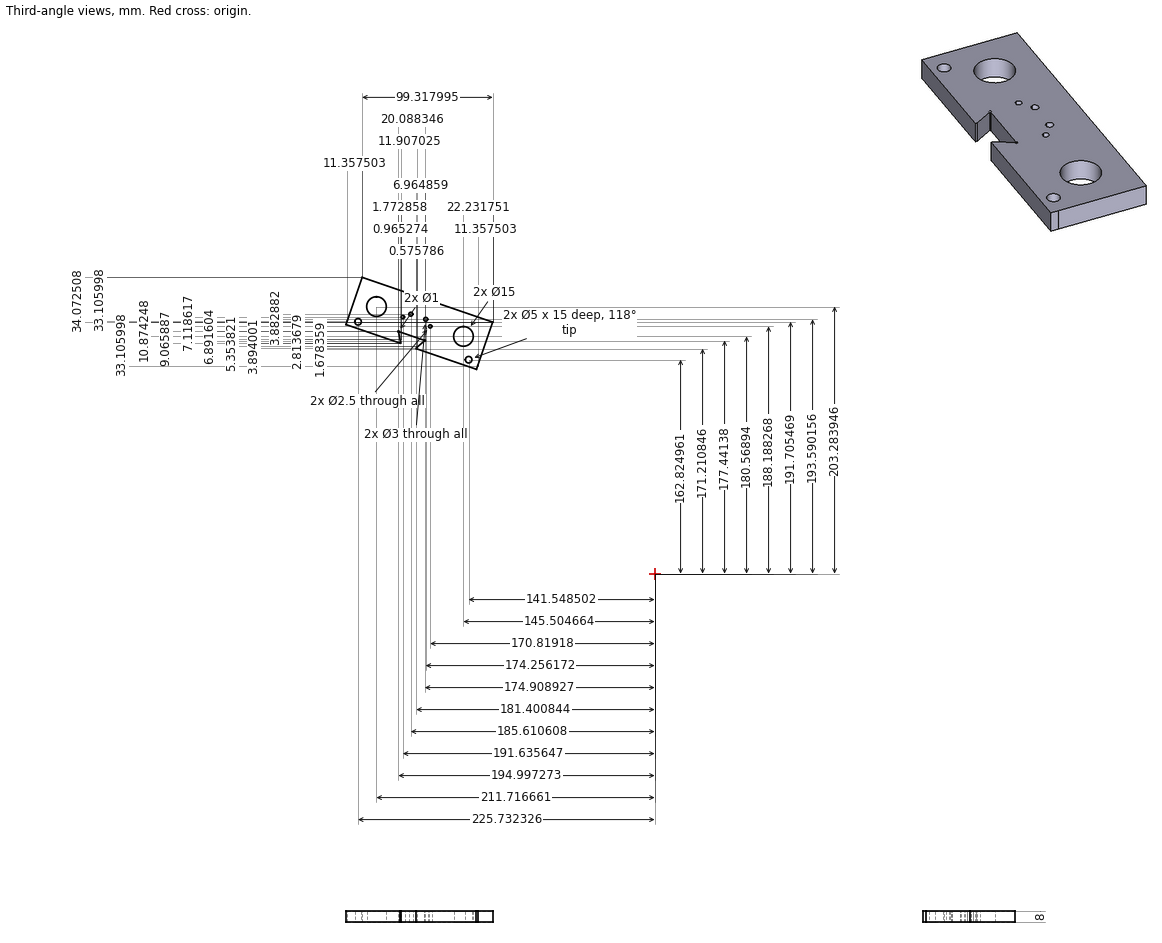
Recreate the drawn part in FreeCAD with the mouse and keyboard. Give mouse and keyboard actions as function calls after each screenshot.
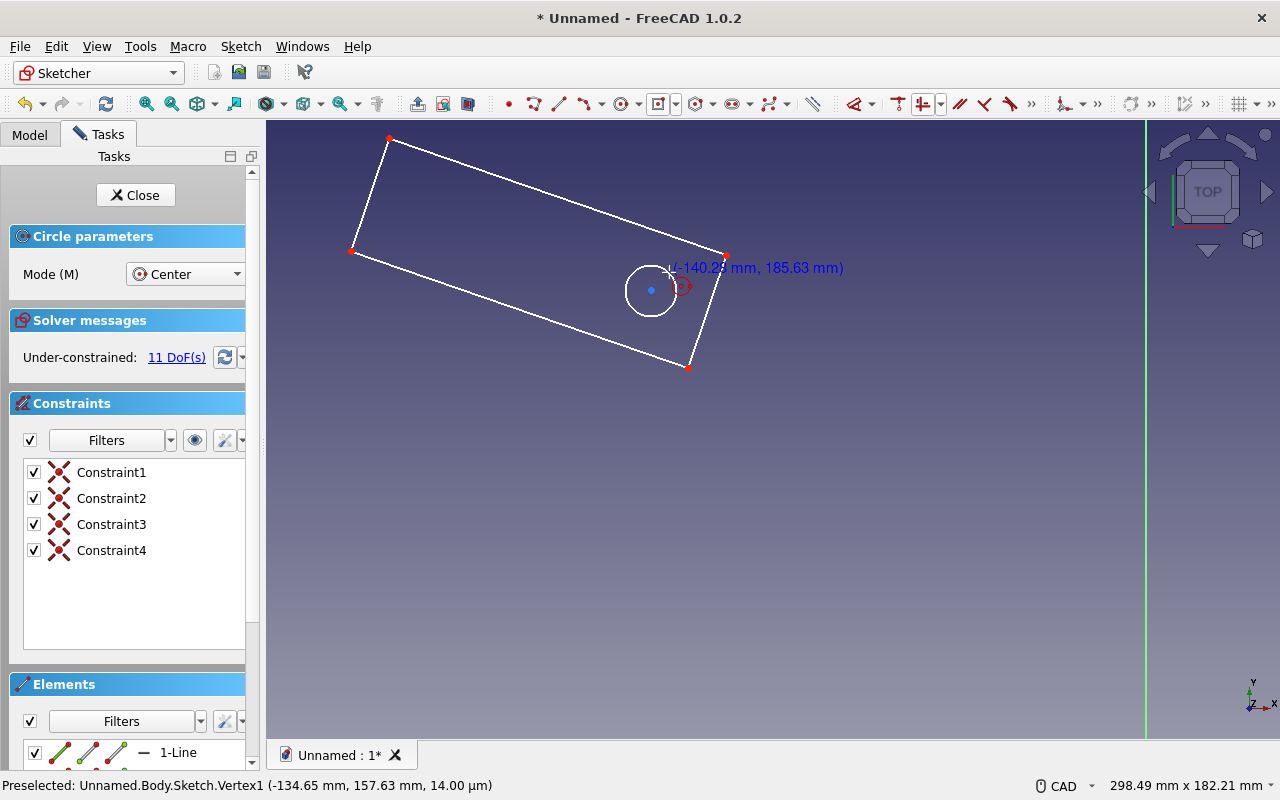
click(426, 213)
click(444, 195)
key(Escape)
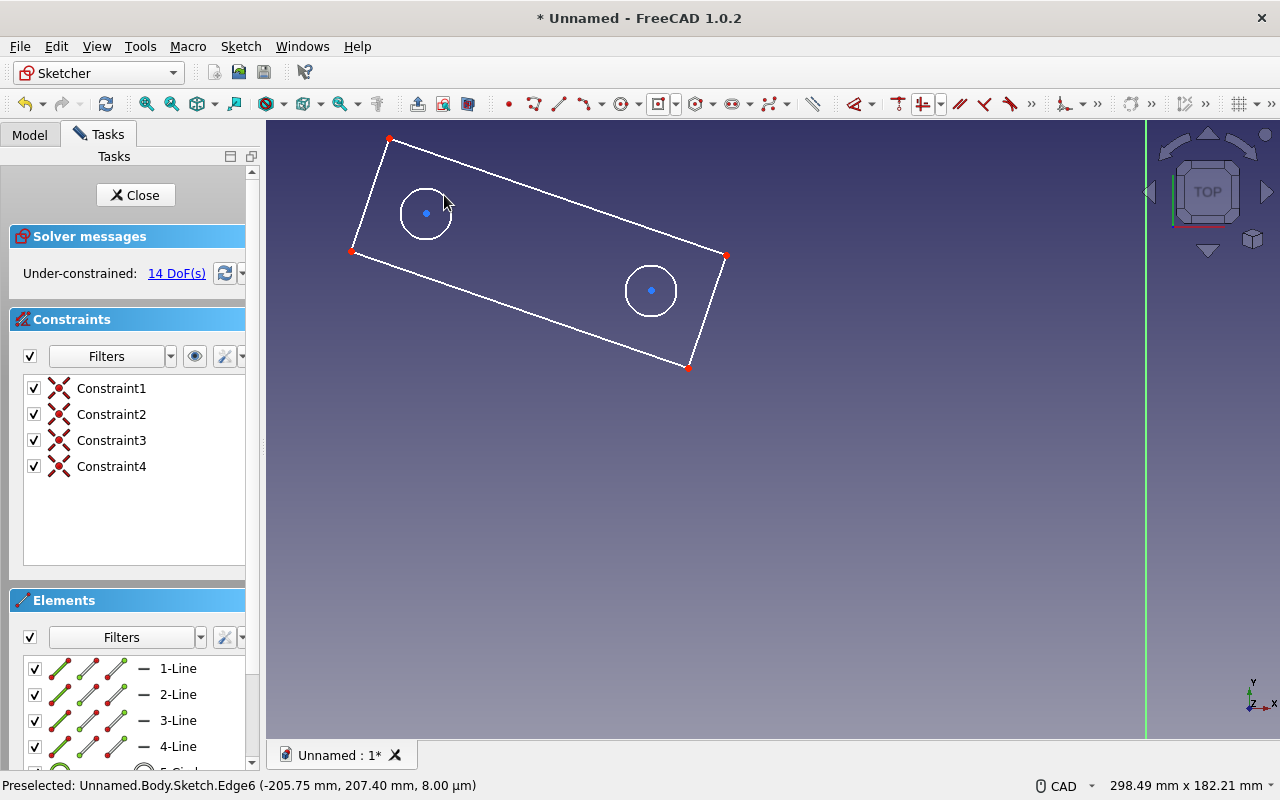
click(669, 273)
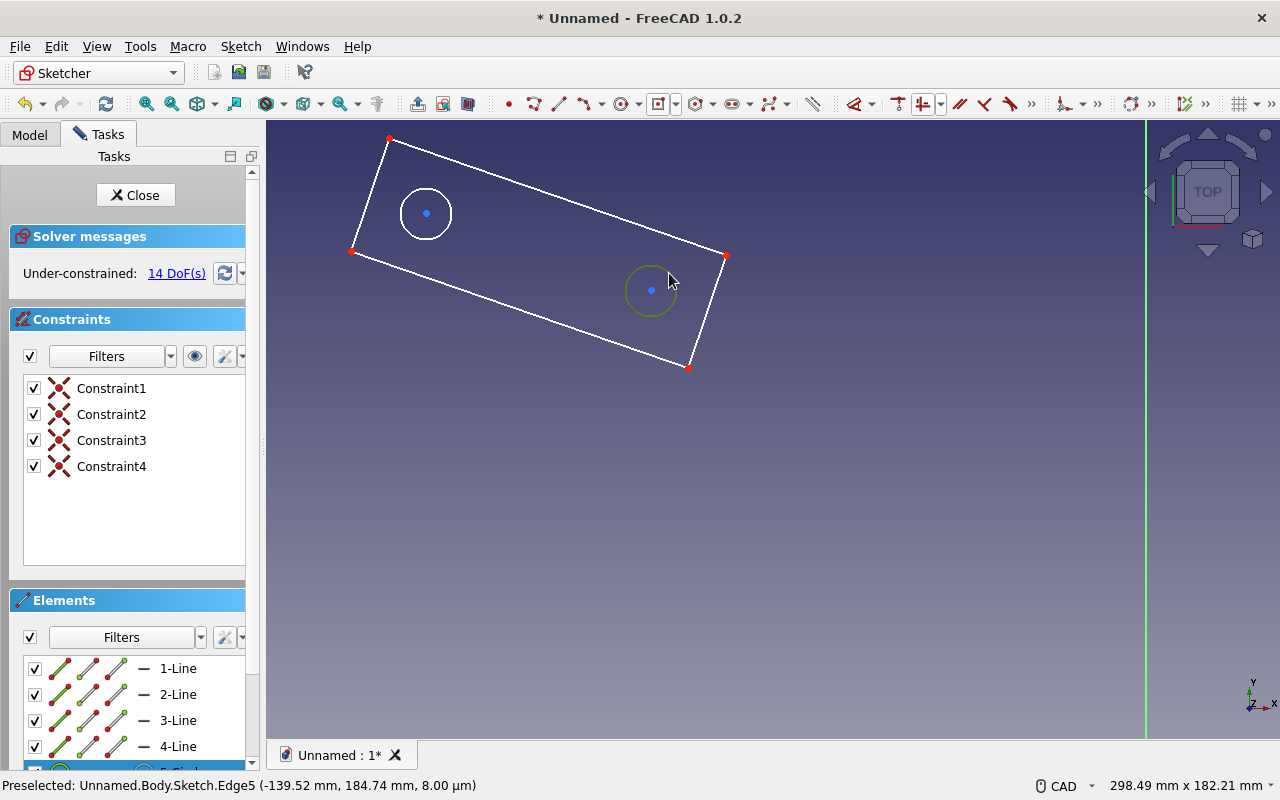
click(444, 196)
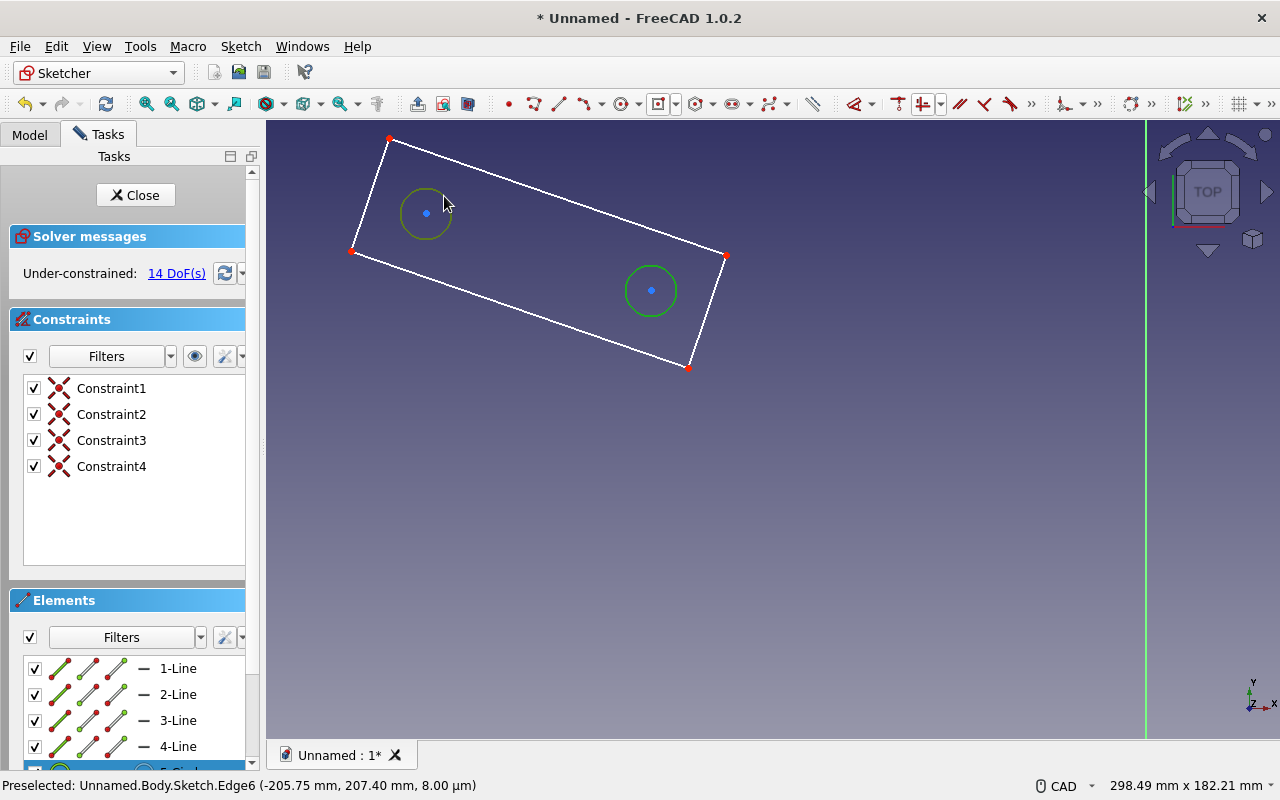
key(e)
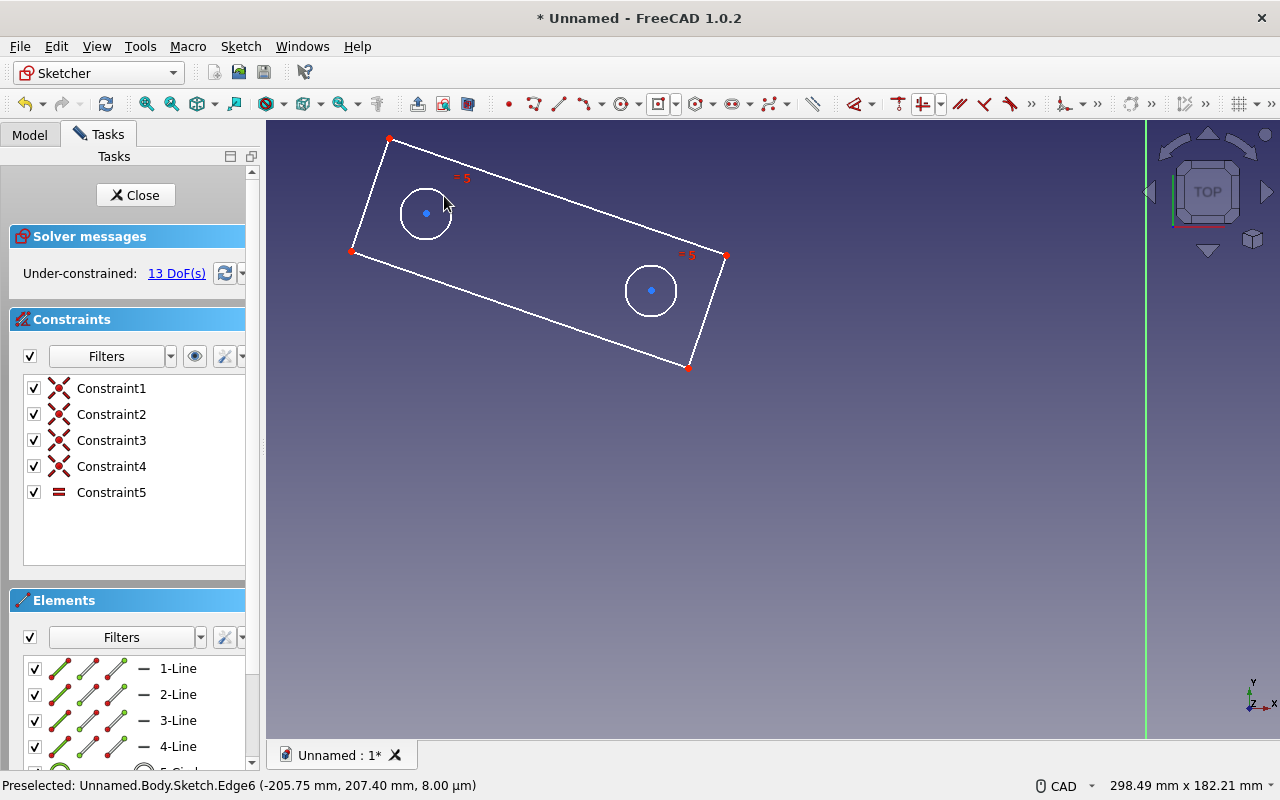
click(669, 273)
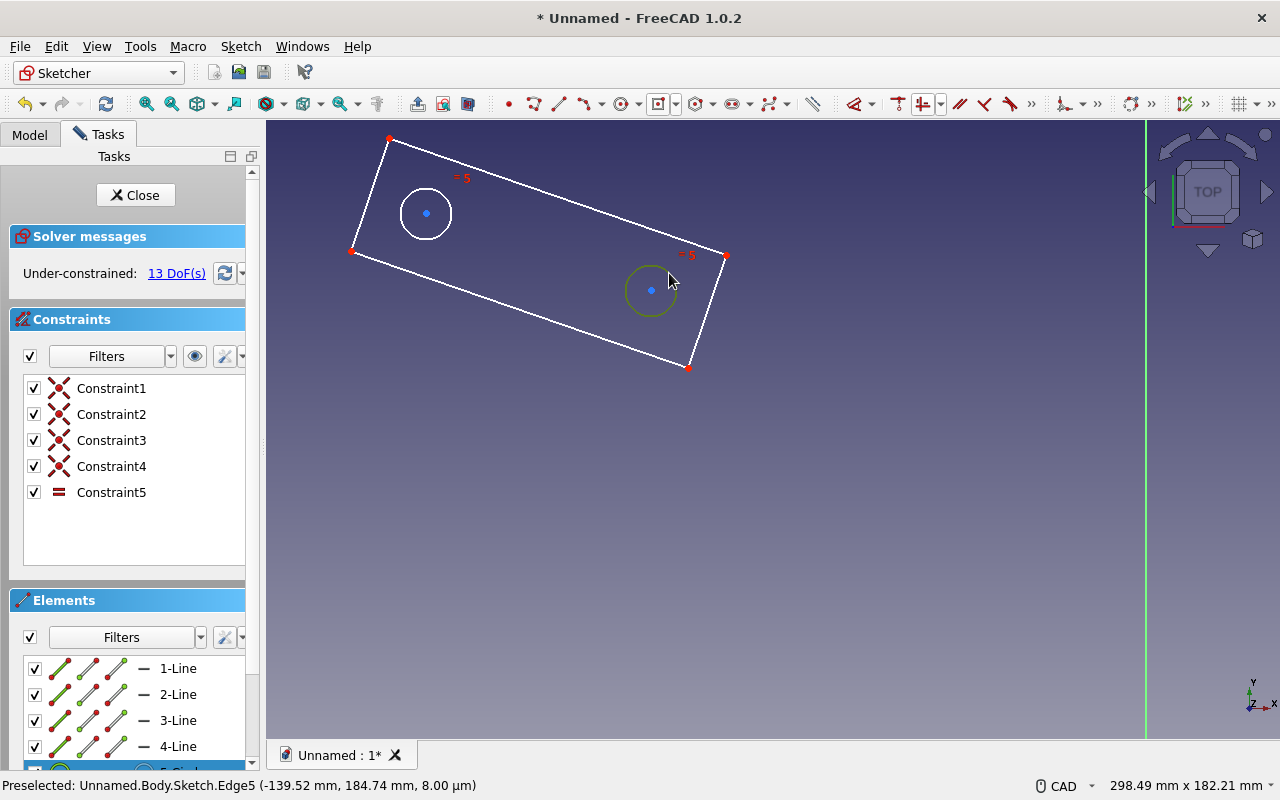
key(k)
key(o)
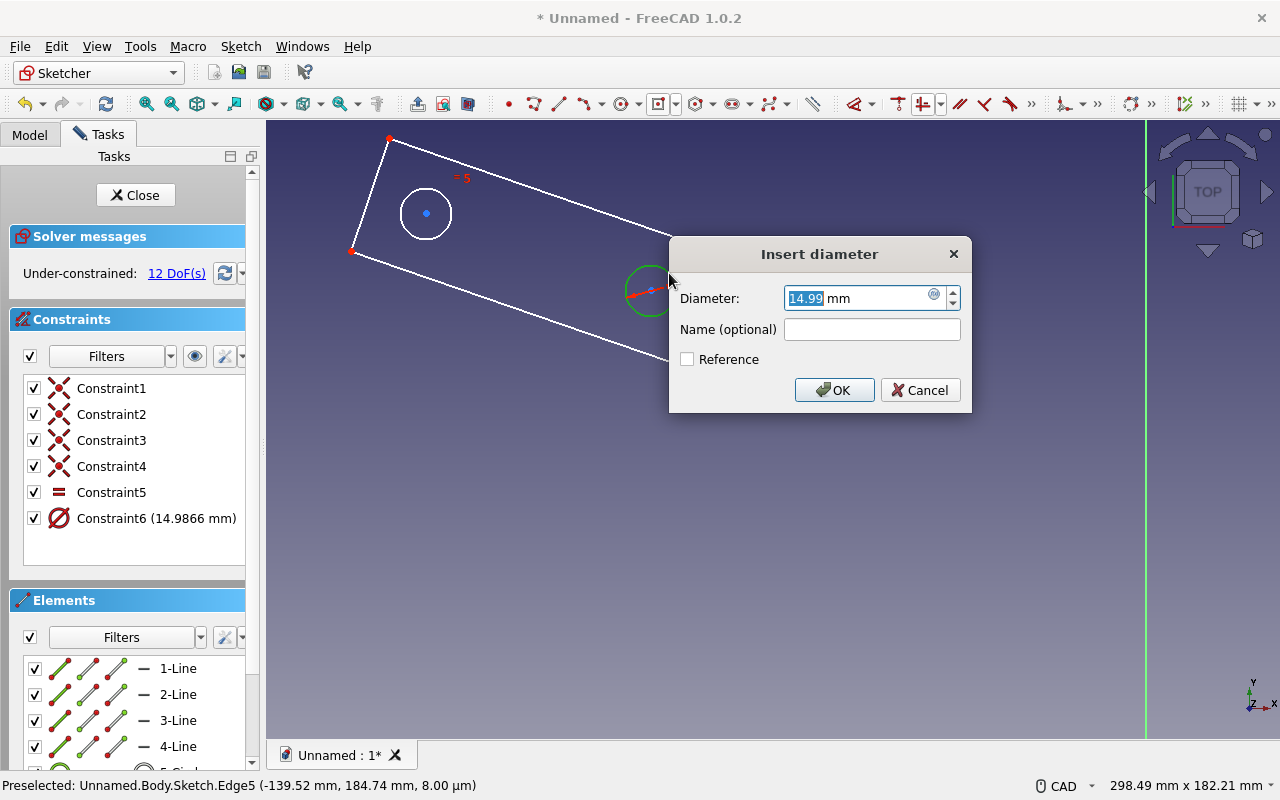
text(15)
key(Return)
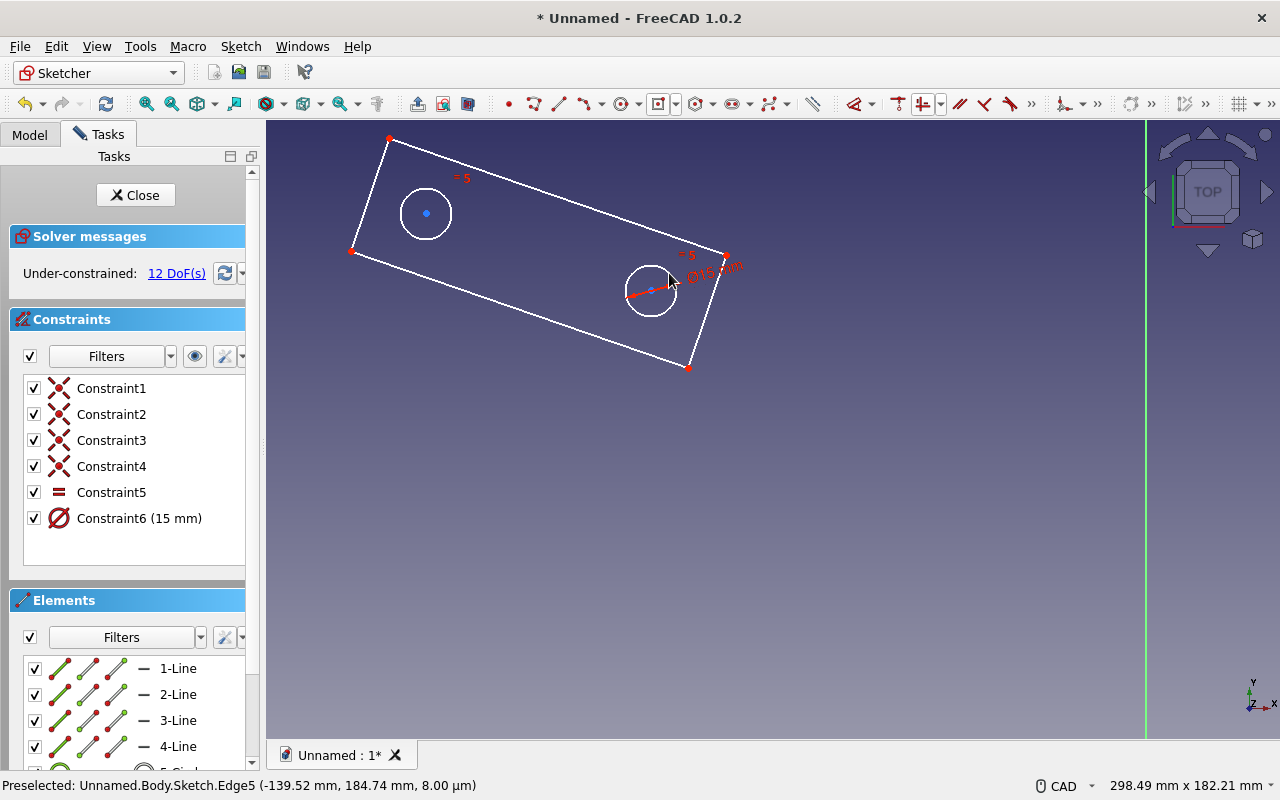
click(651, 291)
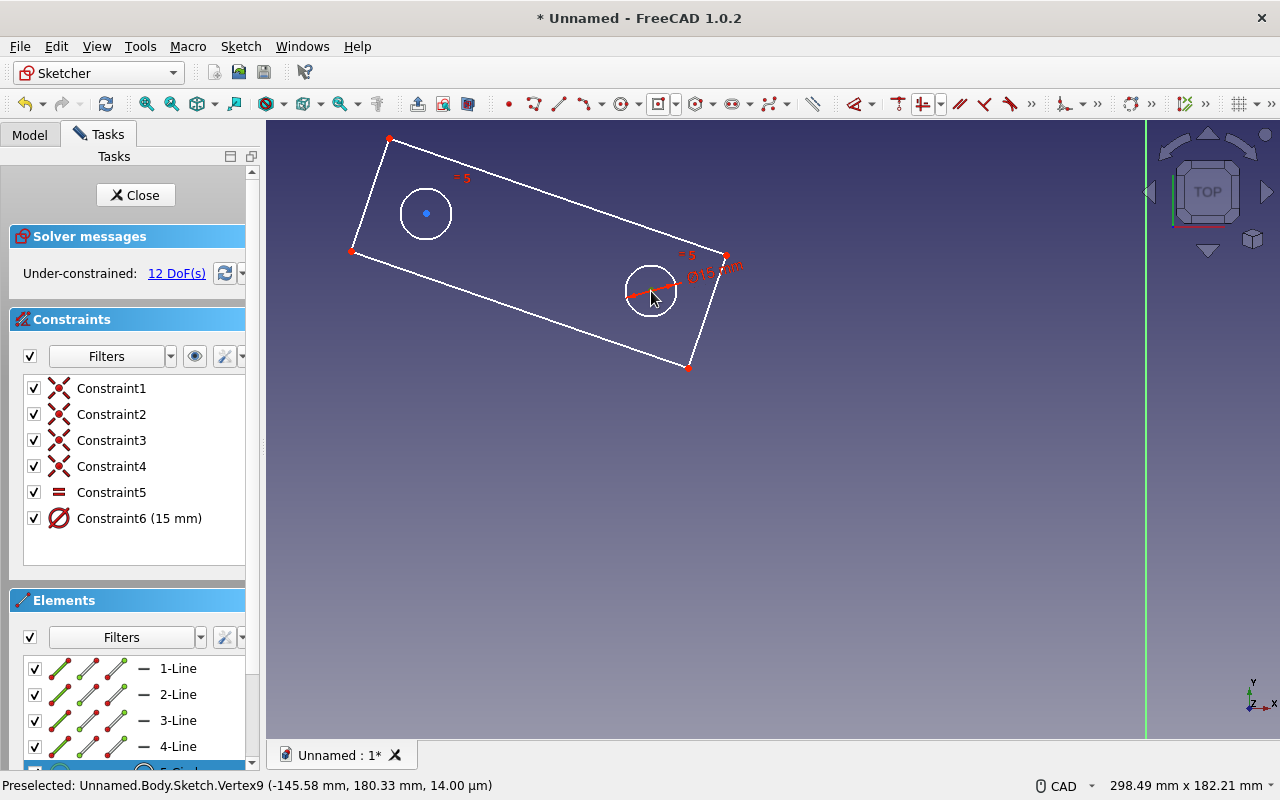
key(i)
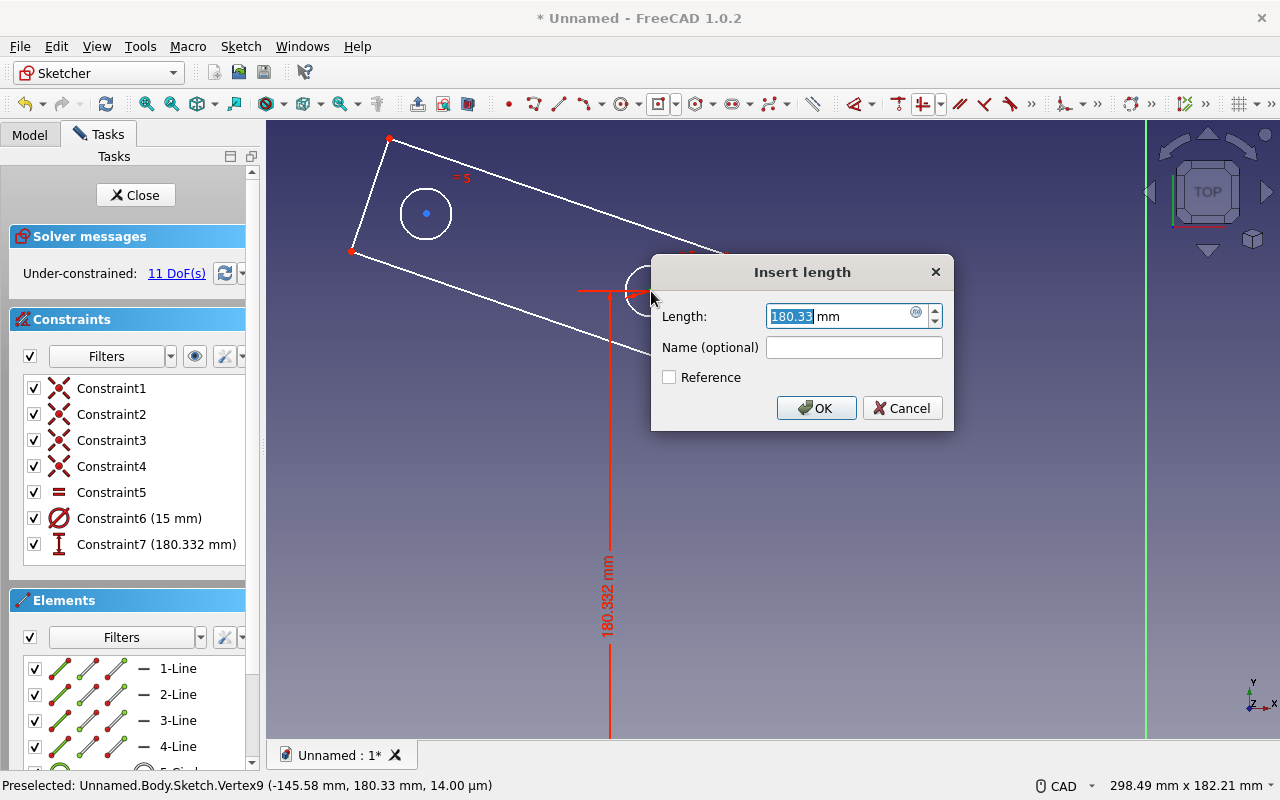
text(180.56894)
key(Return)